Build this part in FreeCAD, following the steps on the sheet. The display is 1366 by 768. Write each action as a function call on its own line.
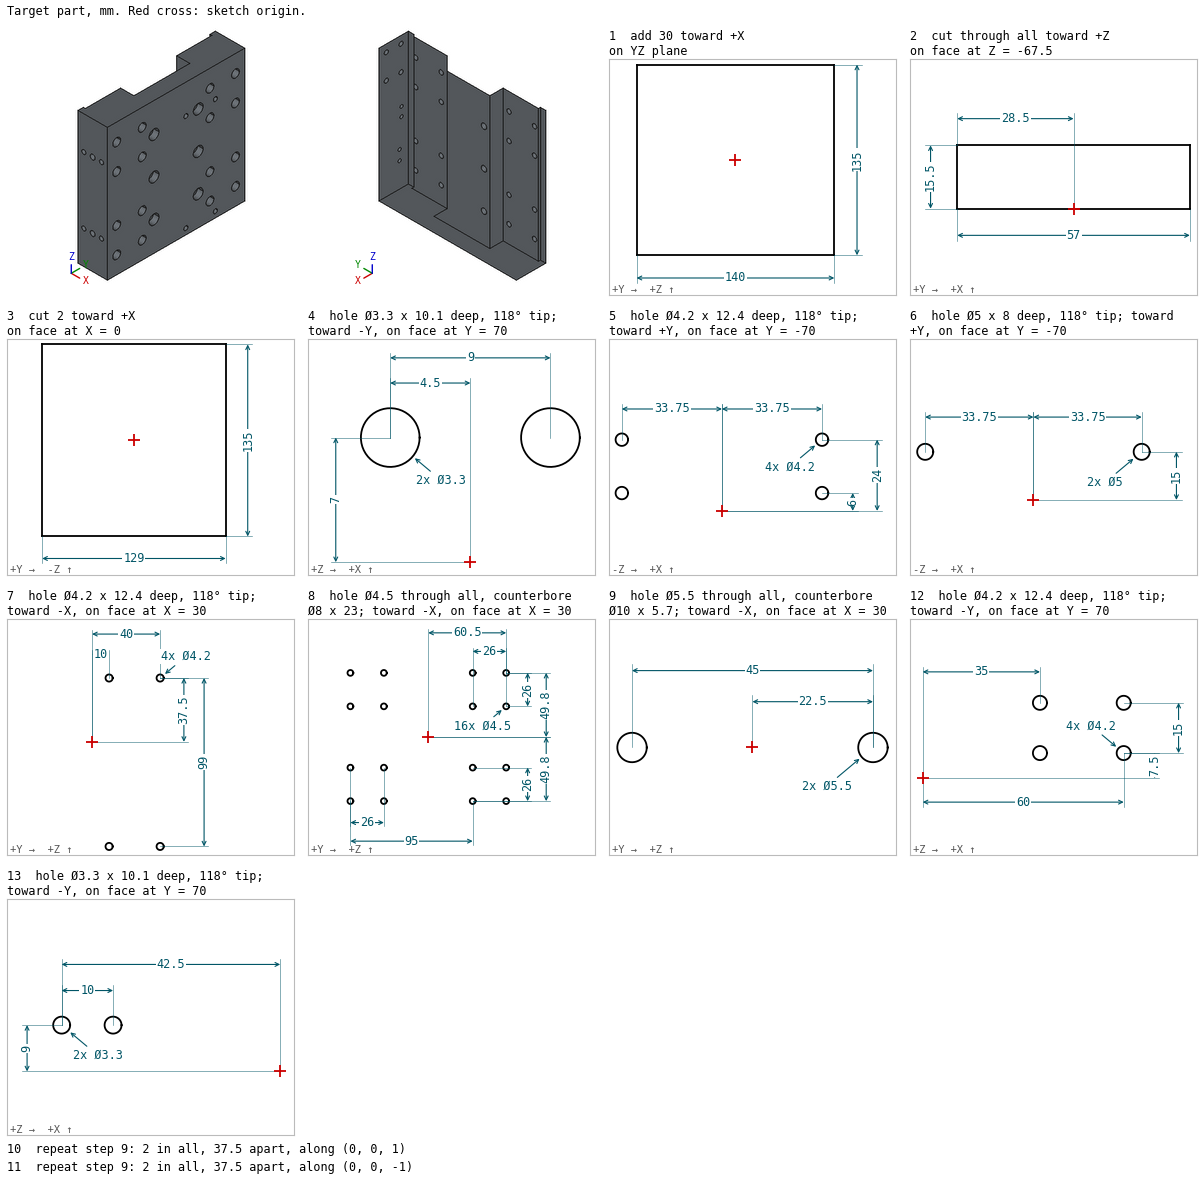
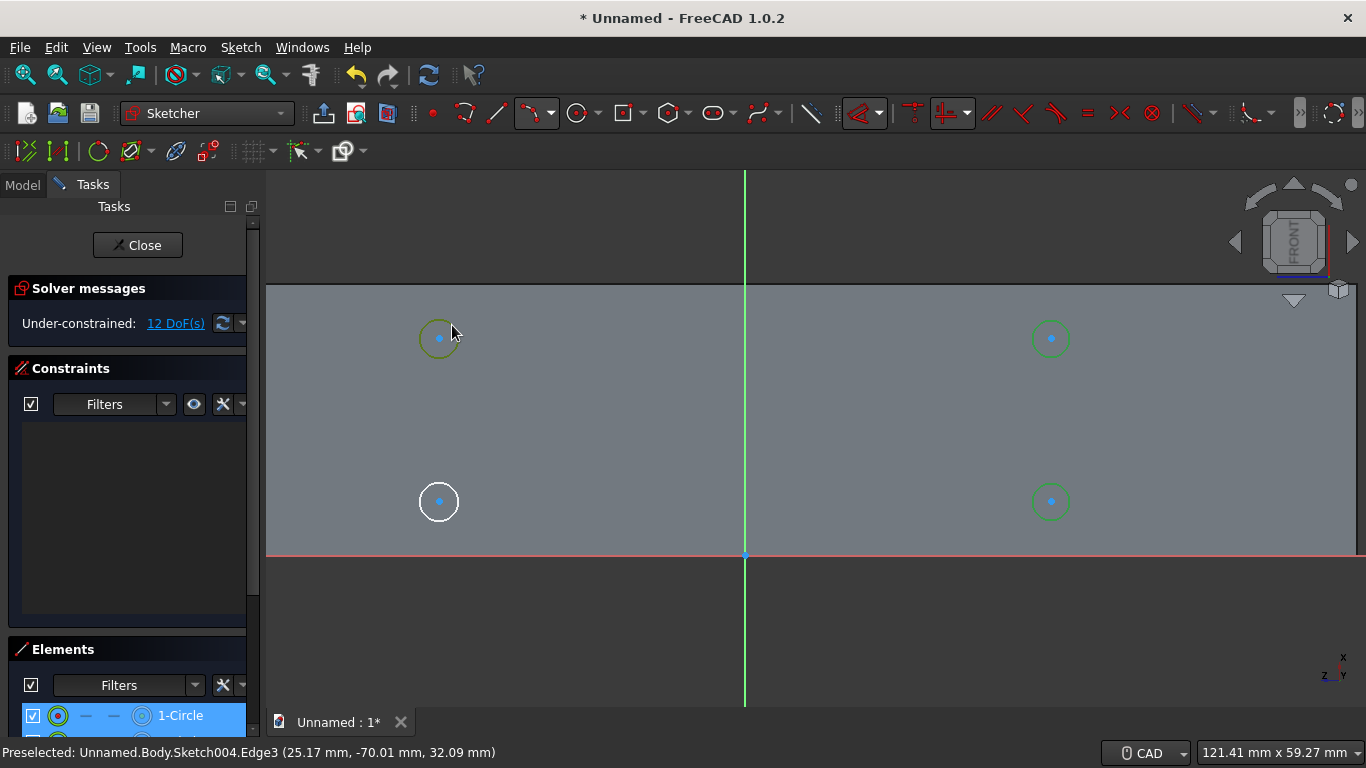
click(452, 488)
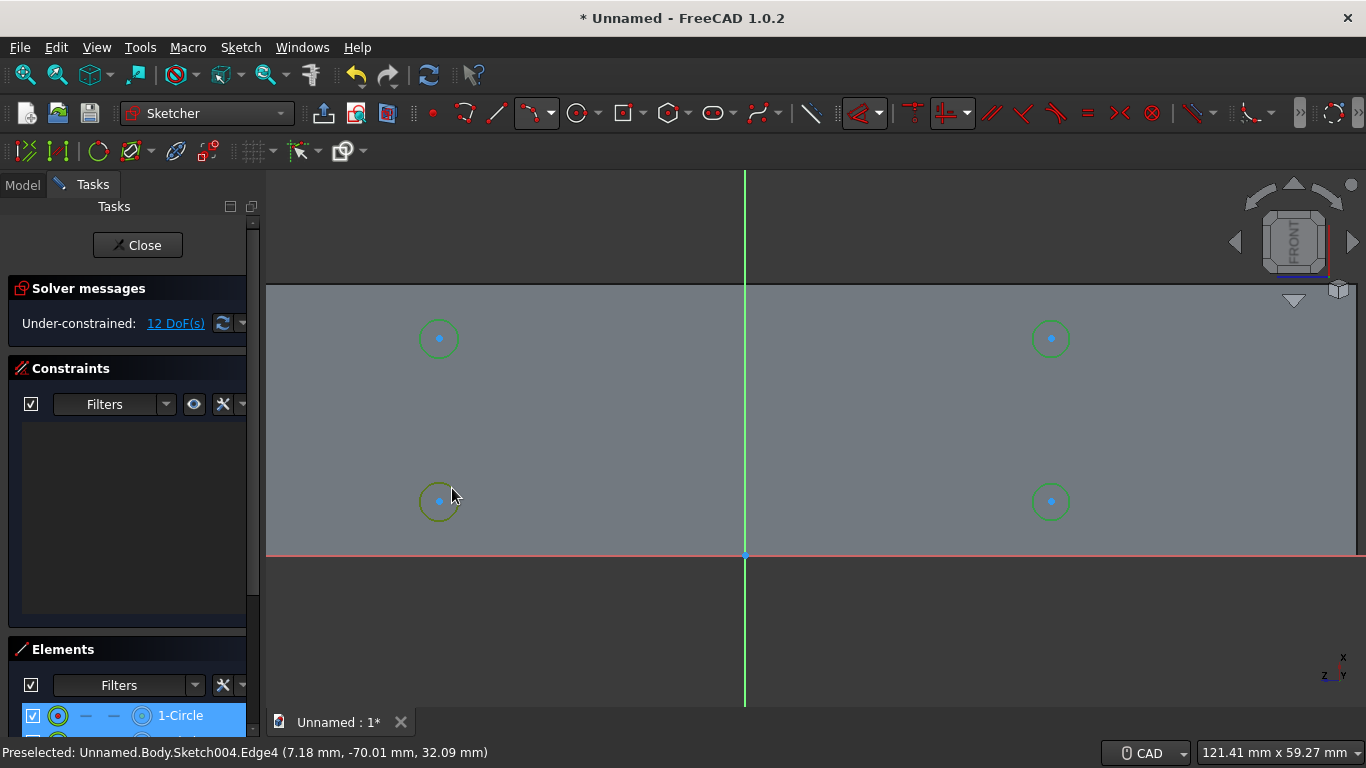
click(1088, 114)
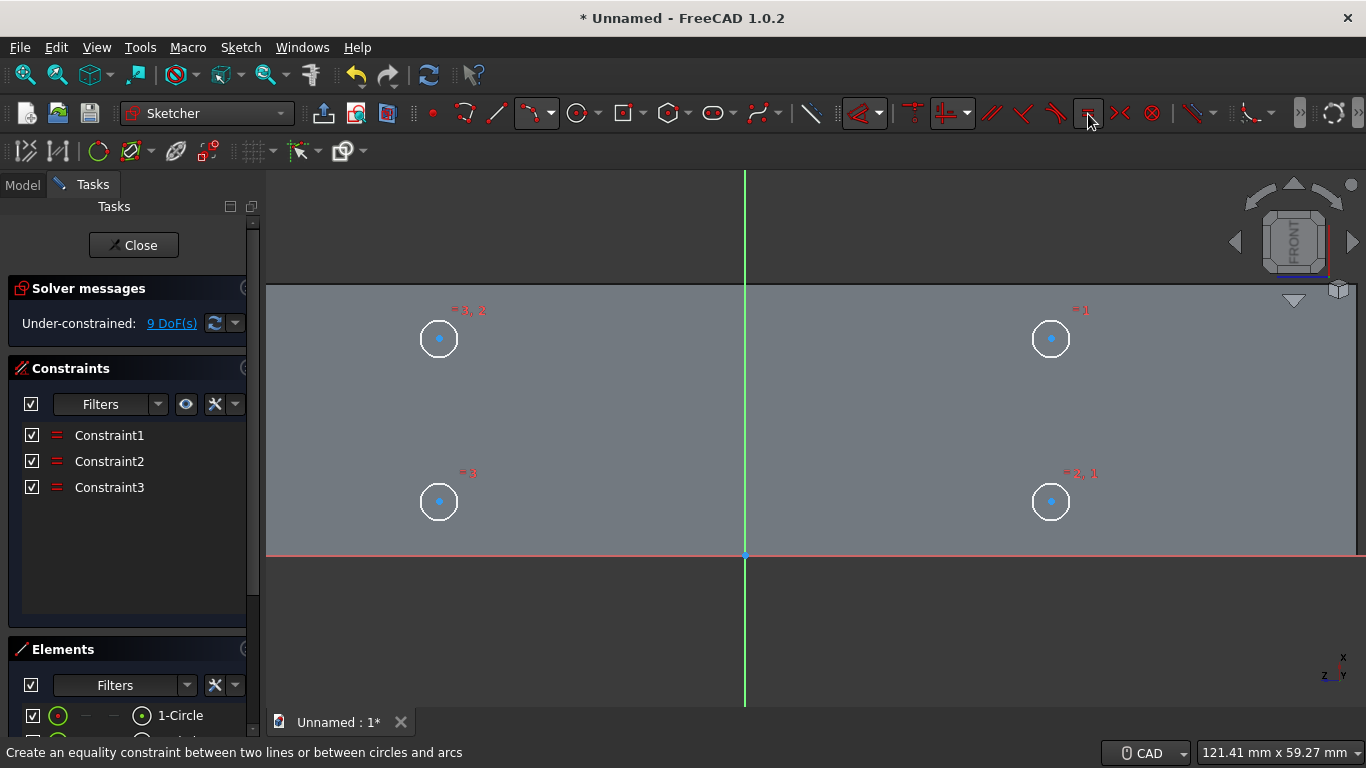
click(1051, 339)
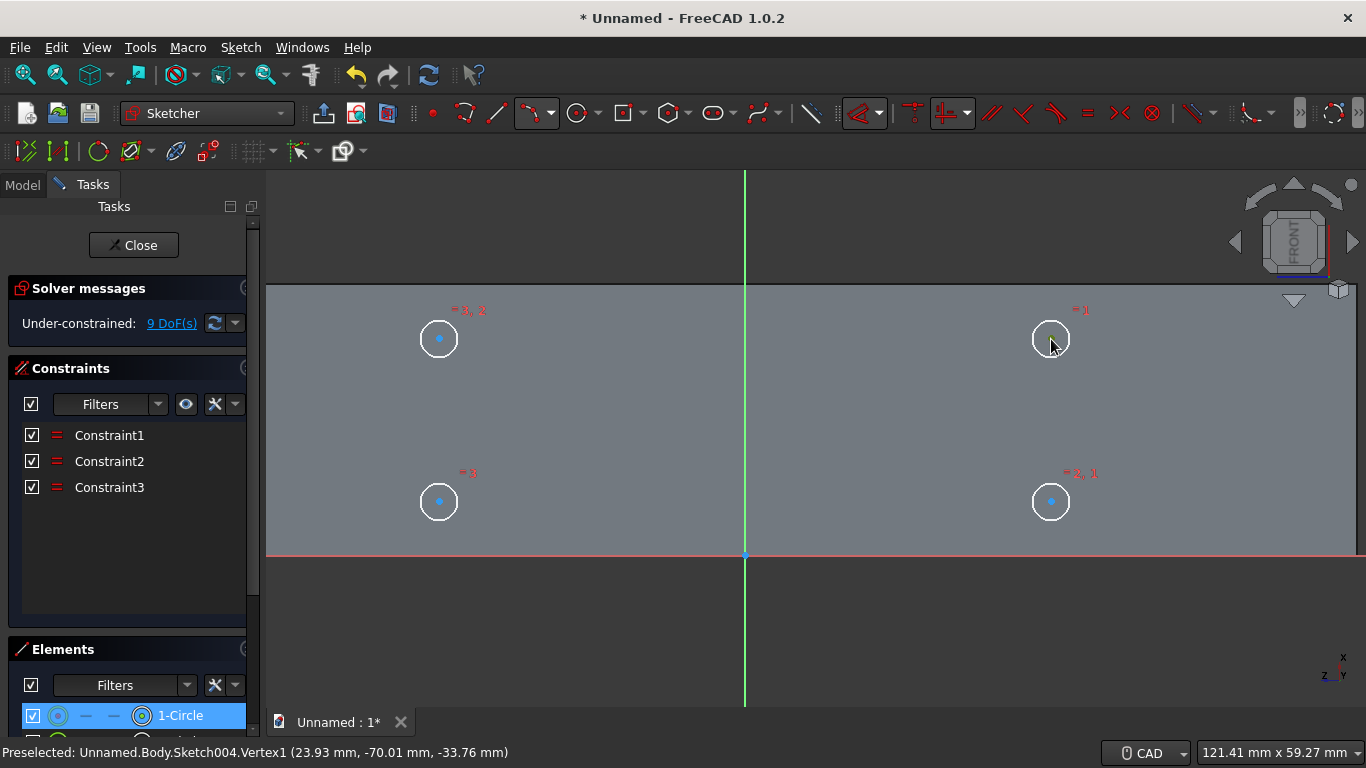
click(1051, 502)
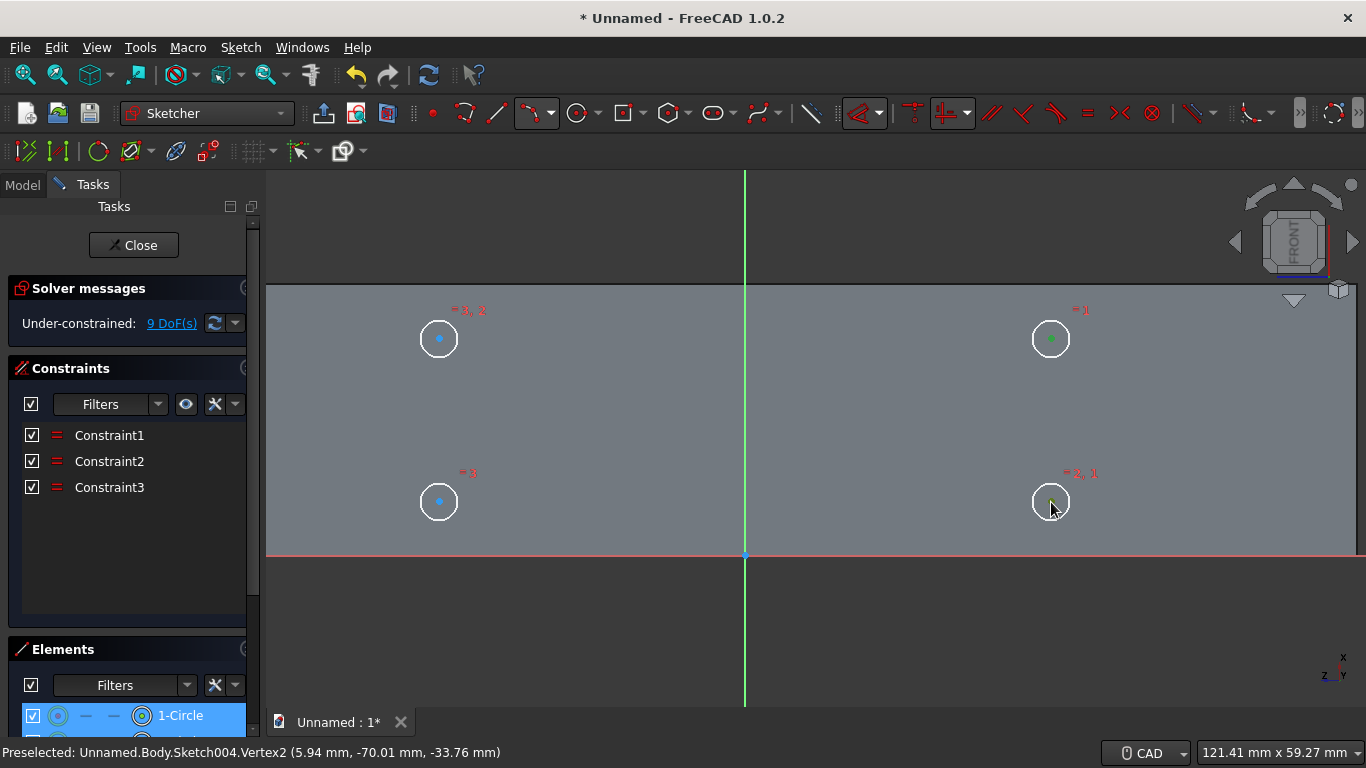
key(v)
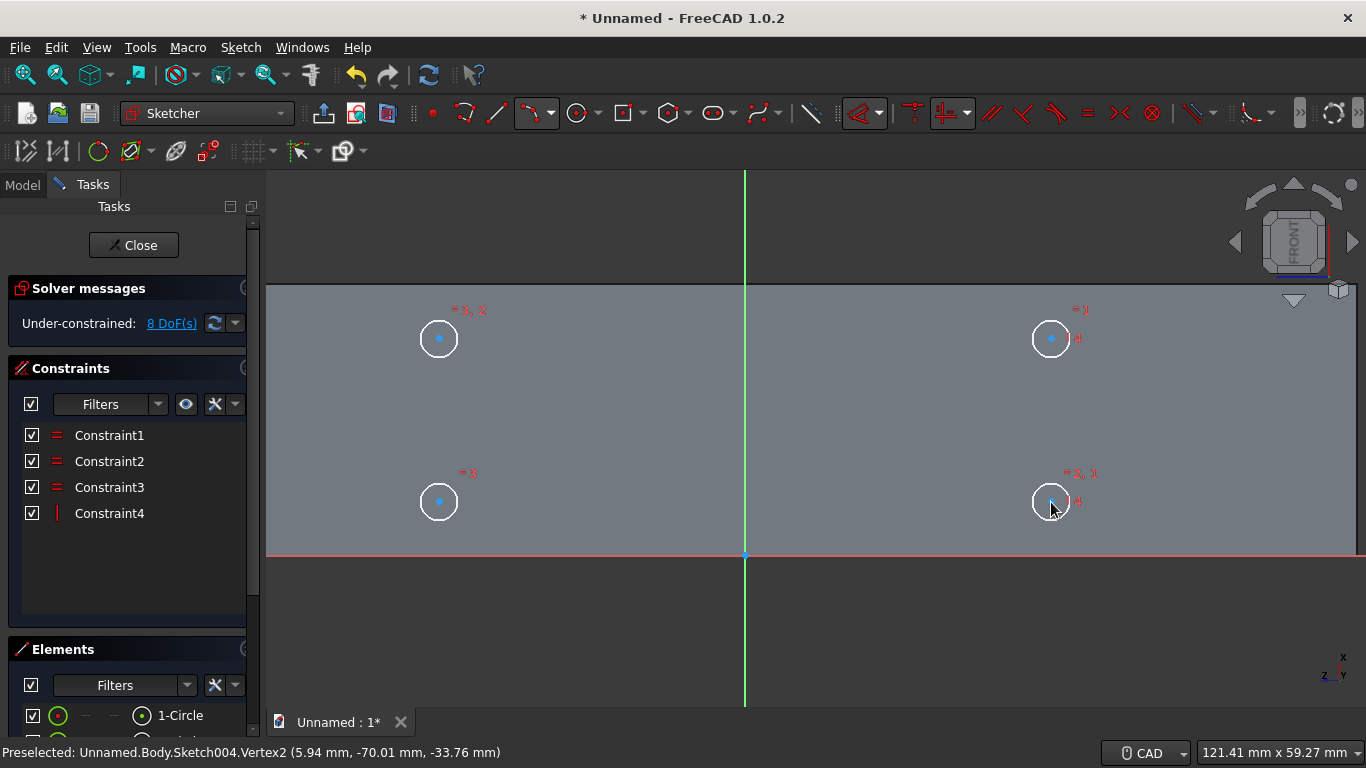
click(1051, 339)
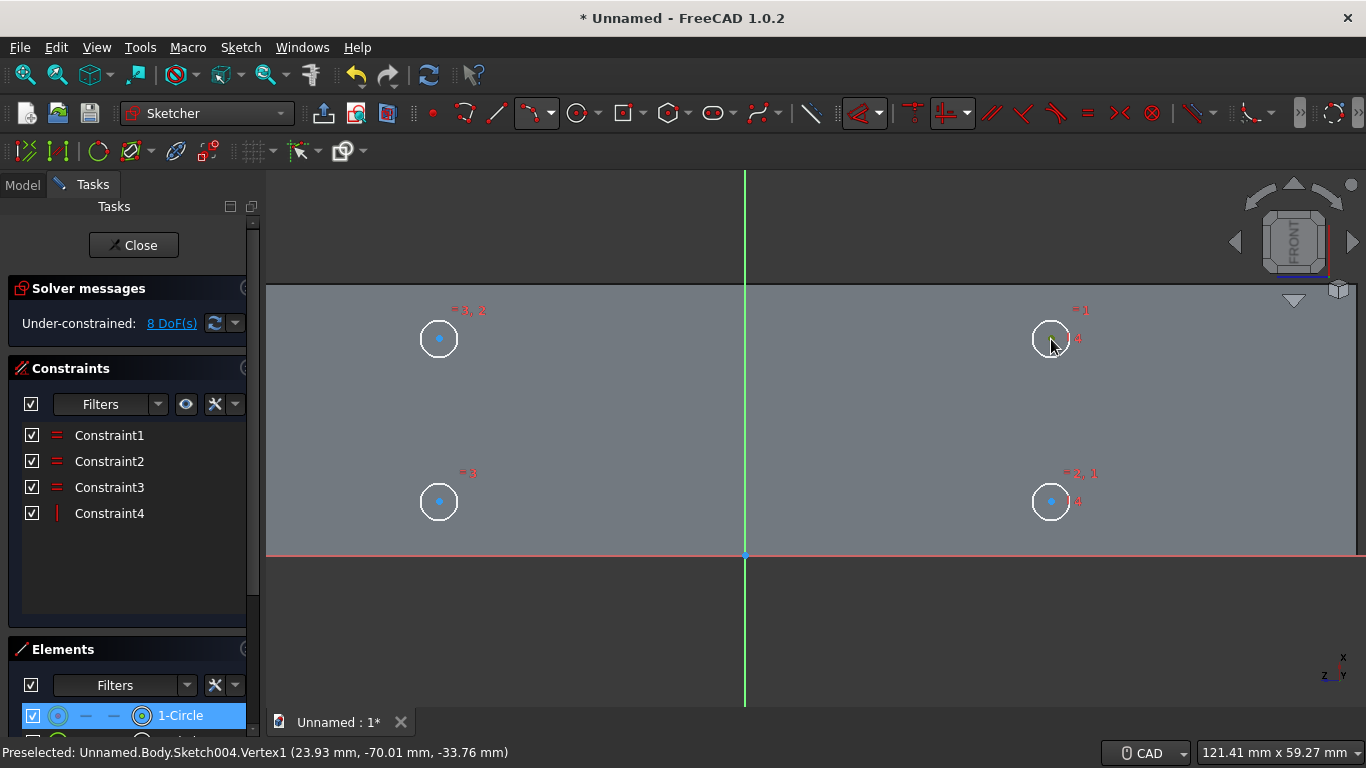
click(439, 339)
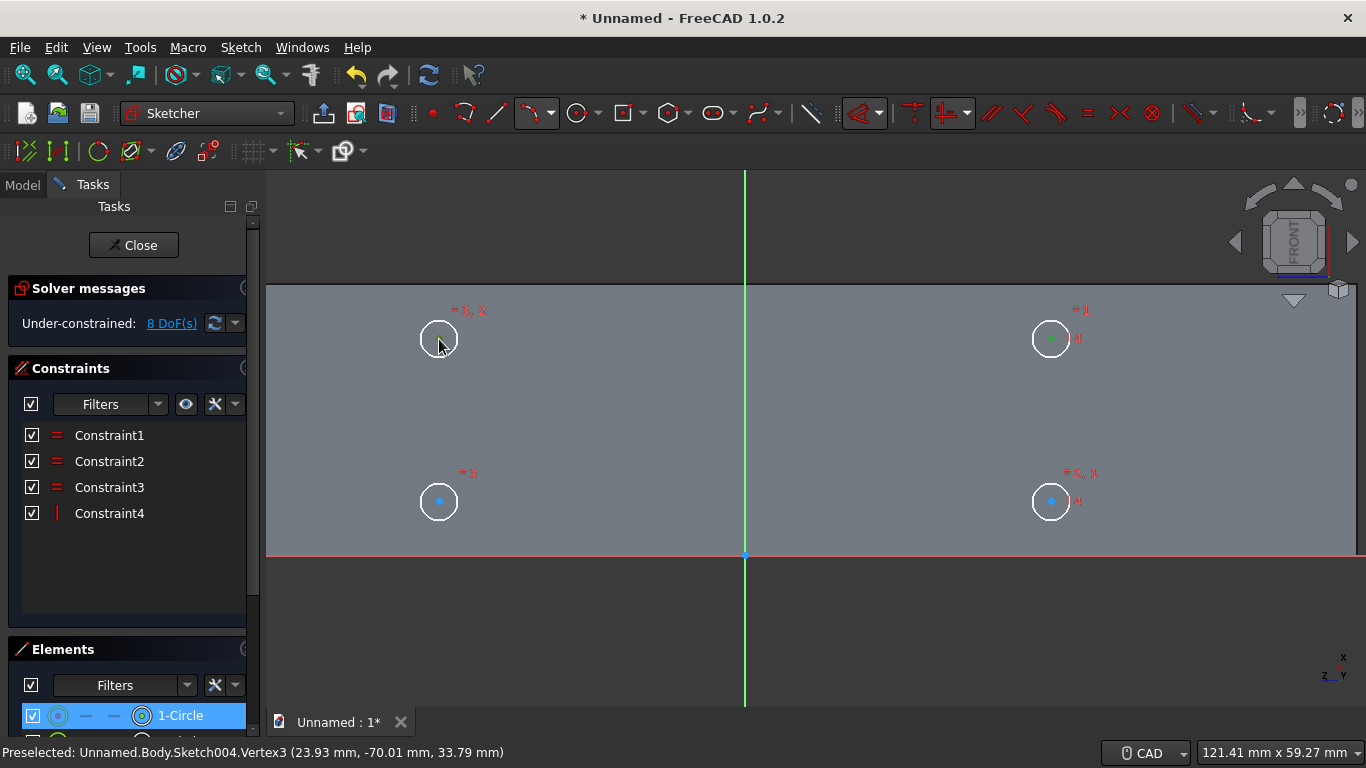
click(970, 114)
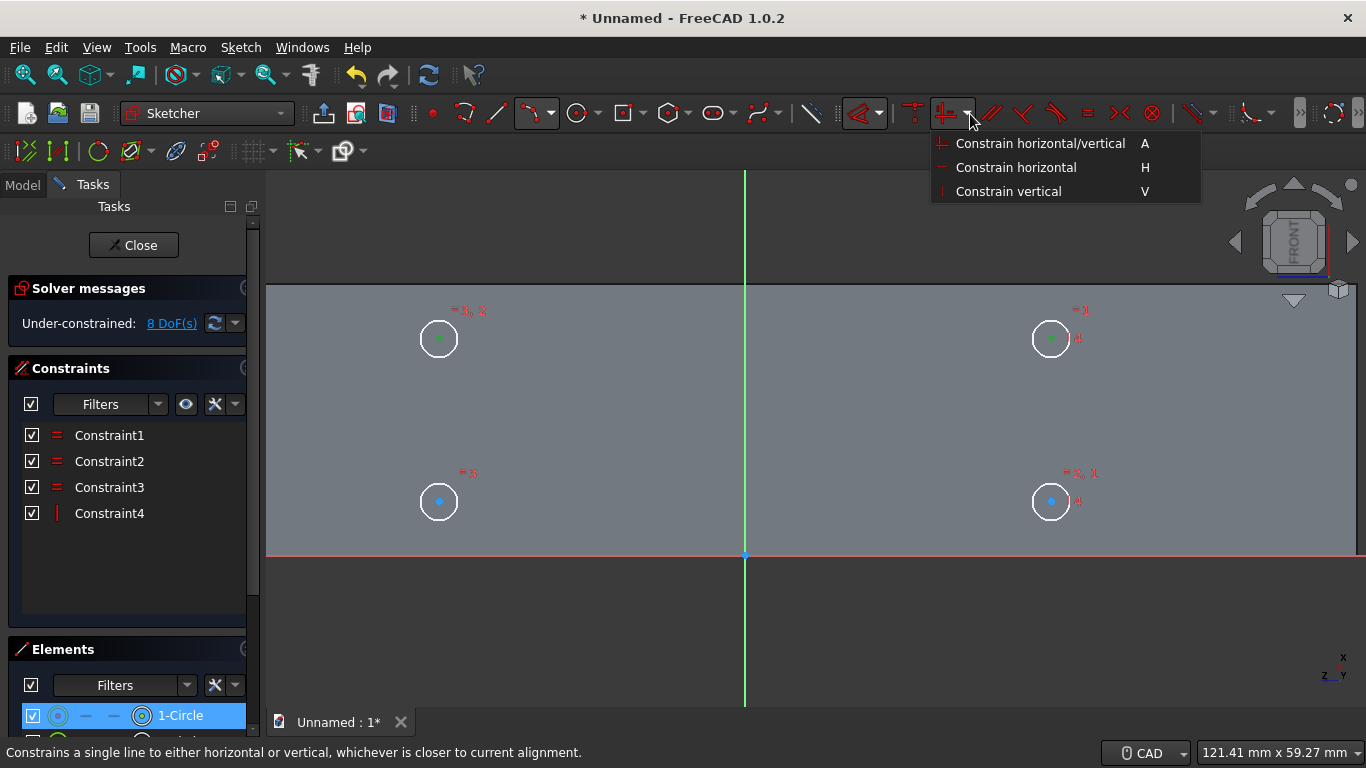
click(1066, 167)